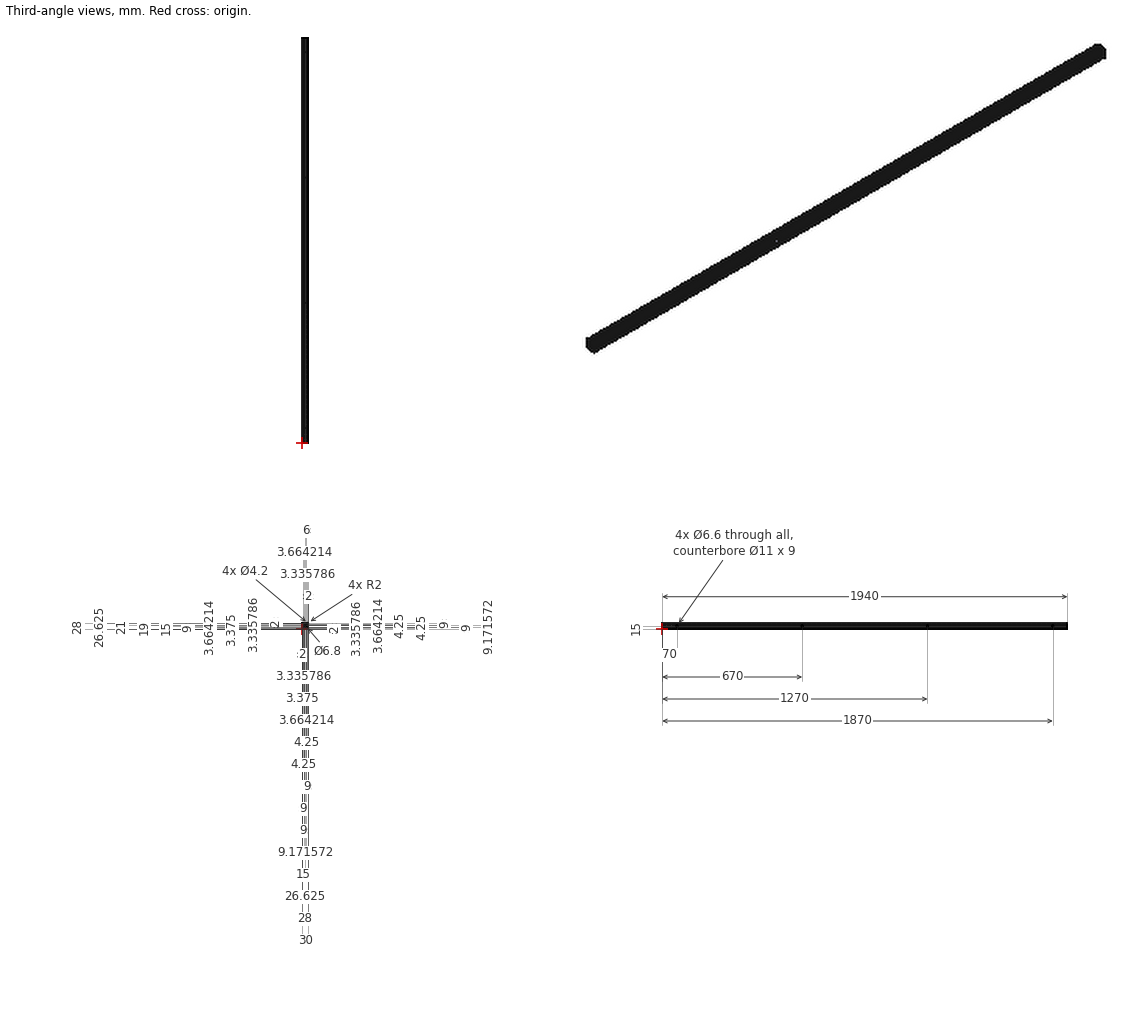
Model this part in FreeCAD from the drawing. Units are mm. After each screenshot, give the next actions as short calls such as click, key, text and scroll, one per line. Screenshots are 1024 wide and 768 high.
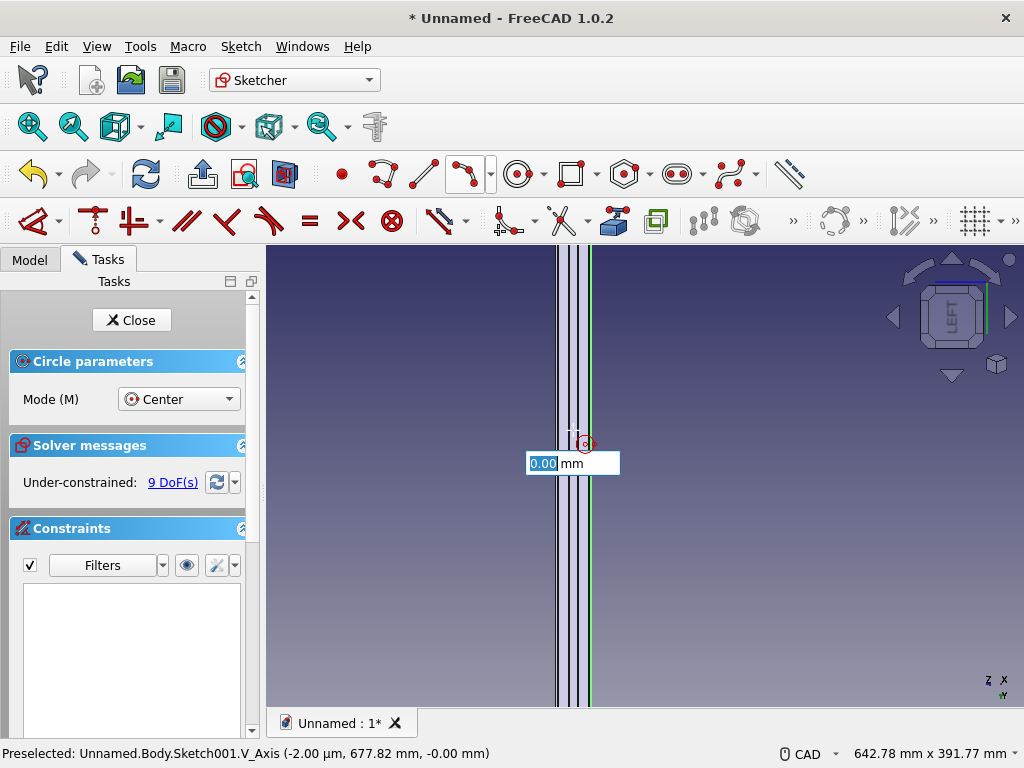
scroll(576, 427, up, 8)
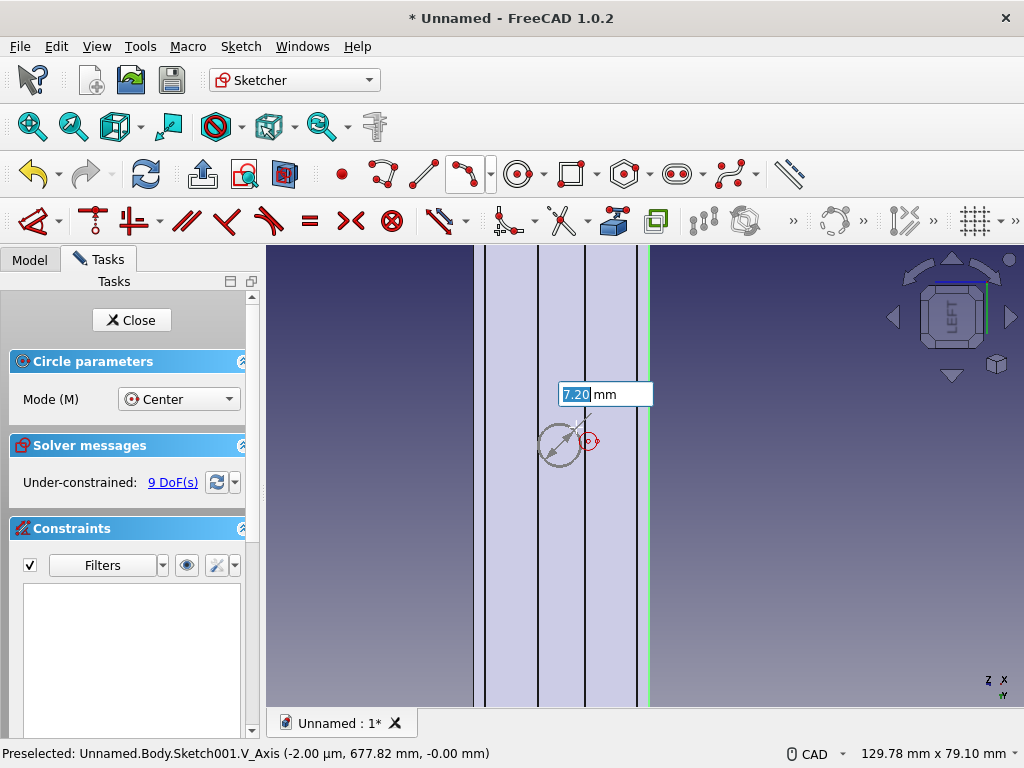
click(575, 424)
key(Escape)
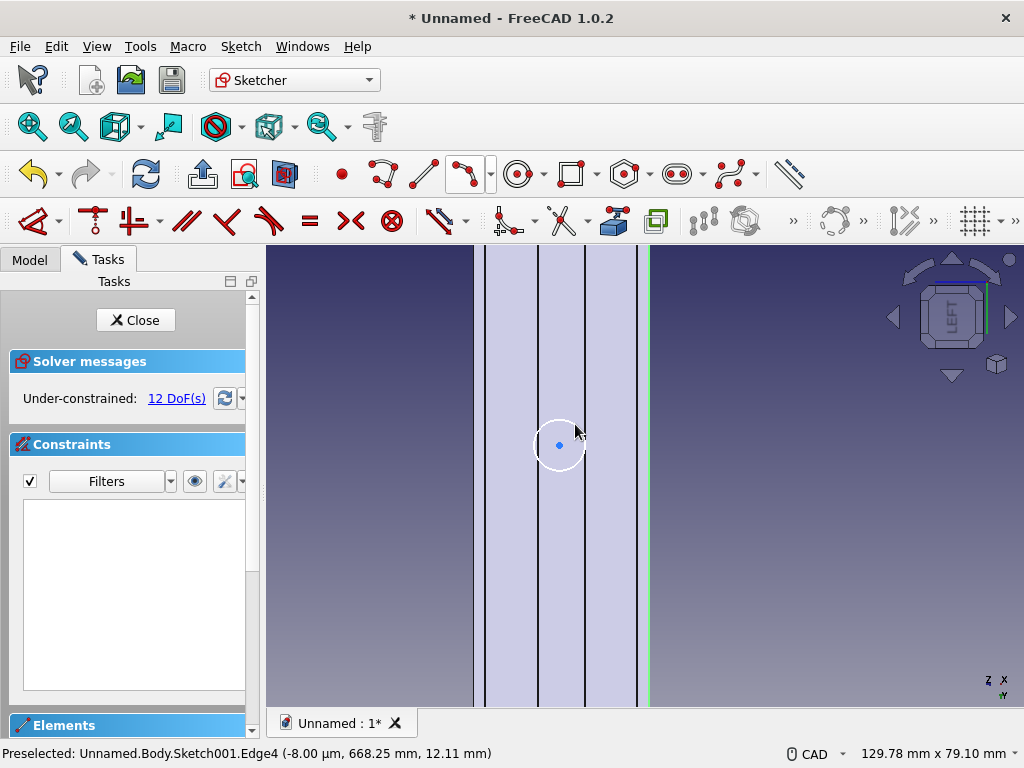
scroll(576, 433, down, 18)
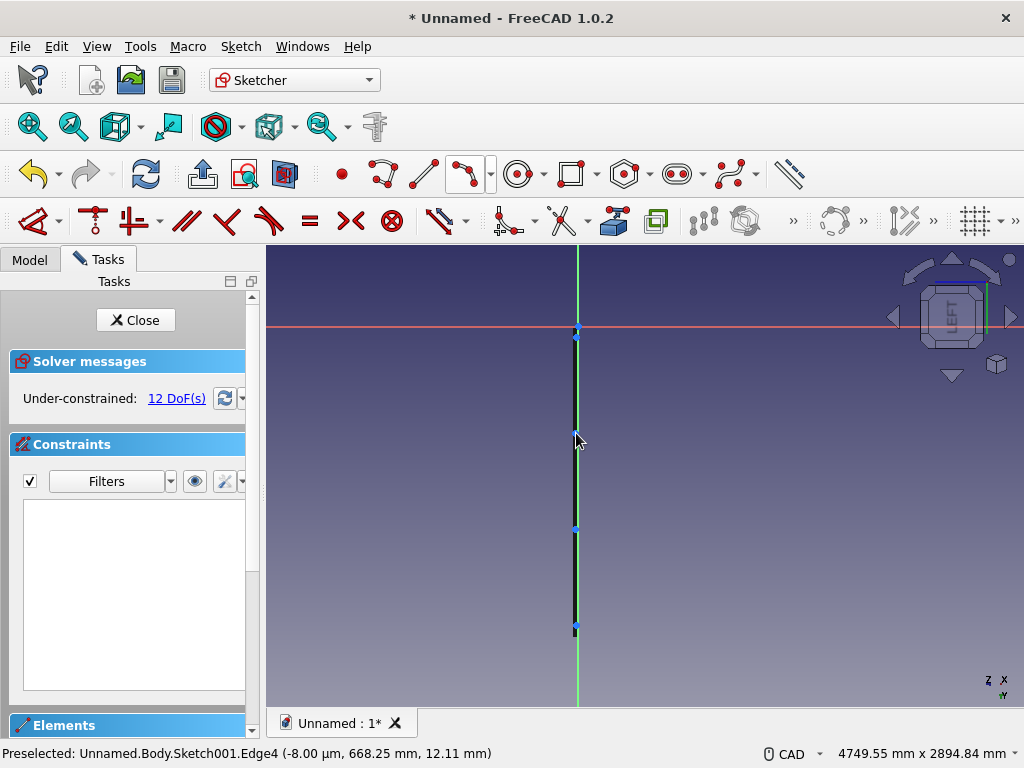
scroll(576, 337, up, 14)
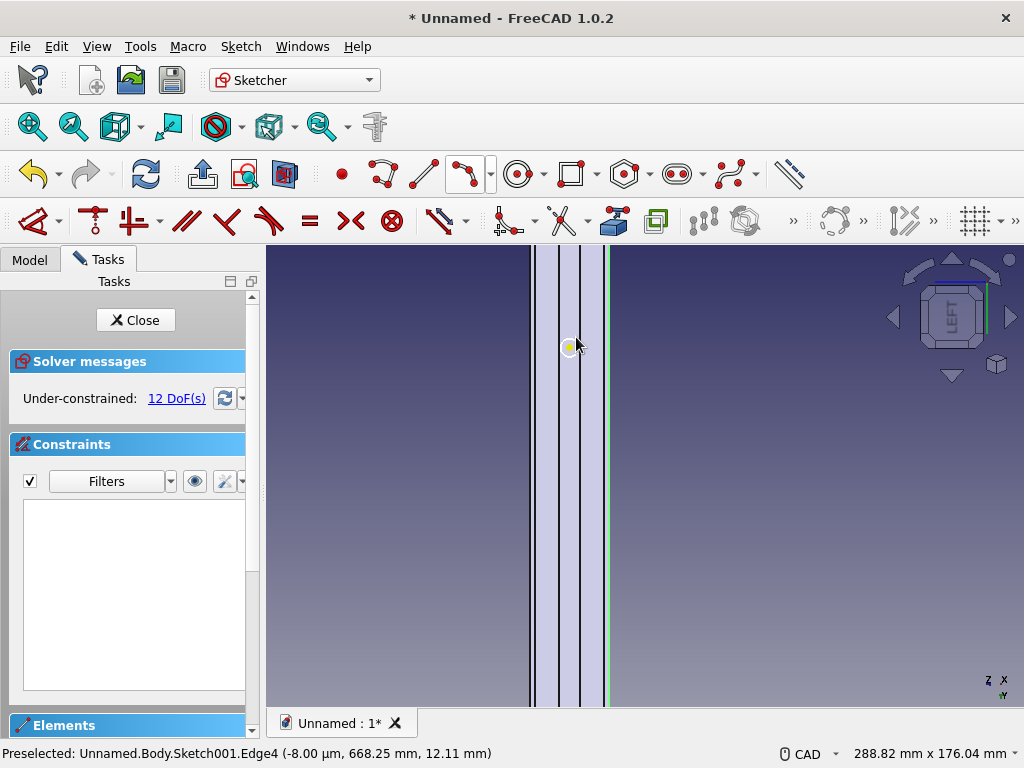
click(576, 341)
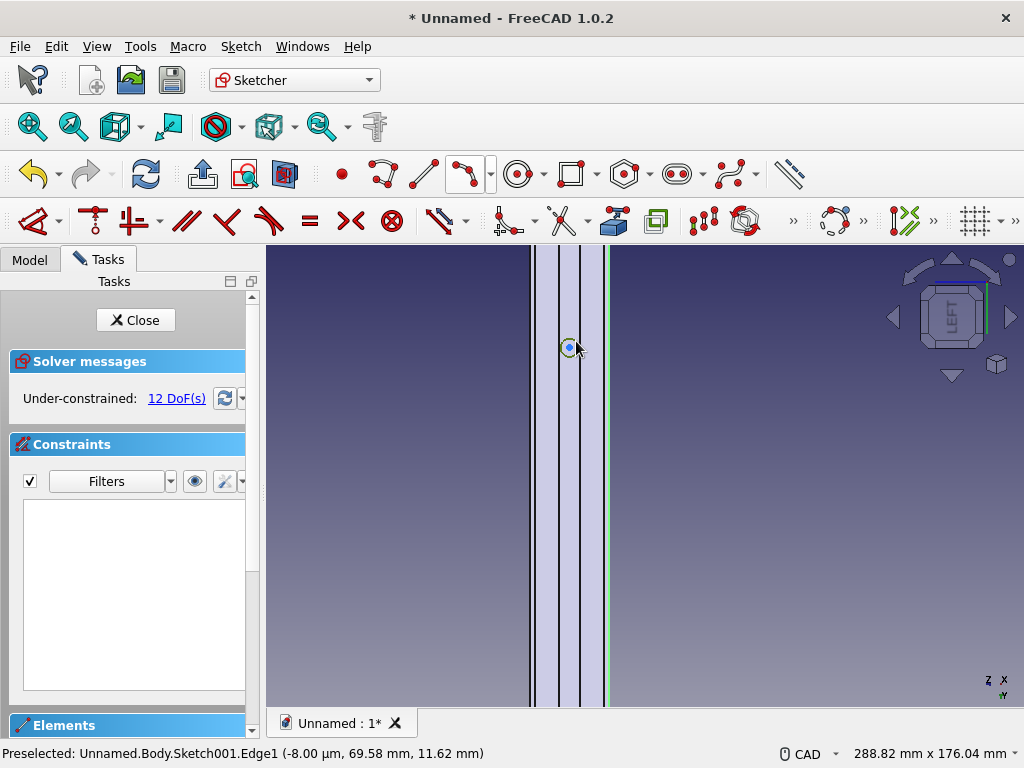
scroll(576, 337, down, 14)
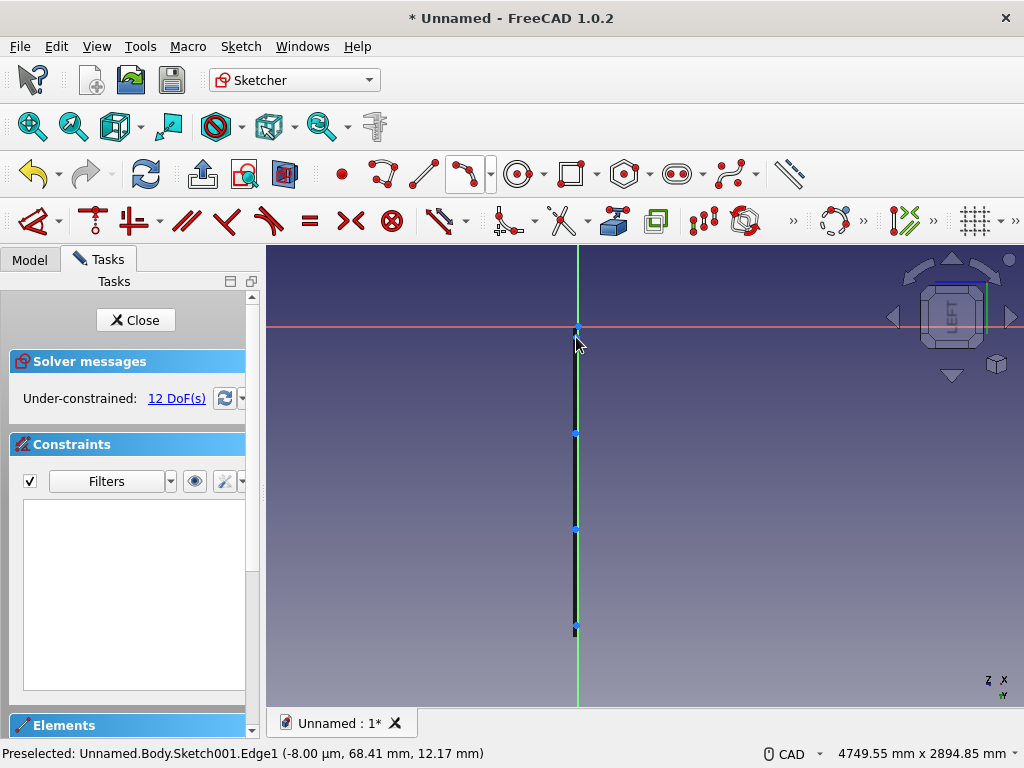
scroll(576, 625, up, 14)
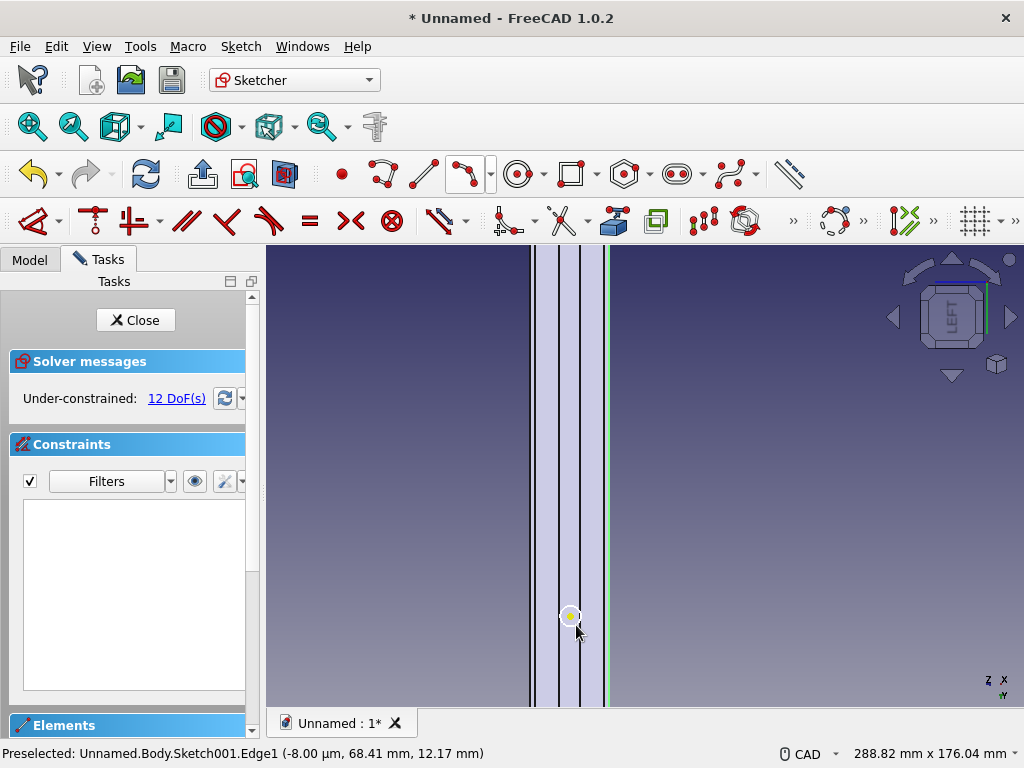
click(578, 609)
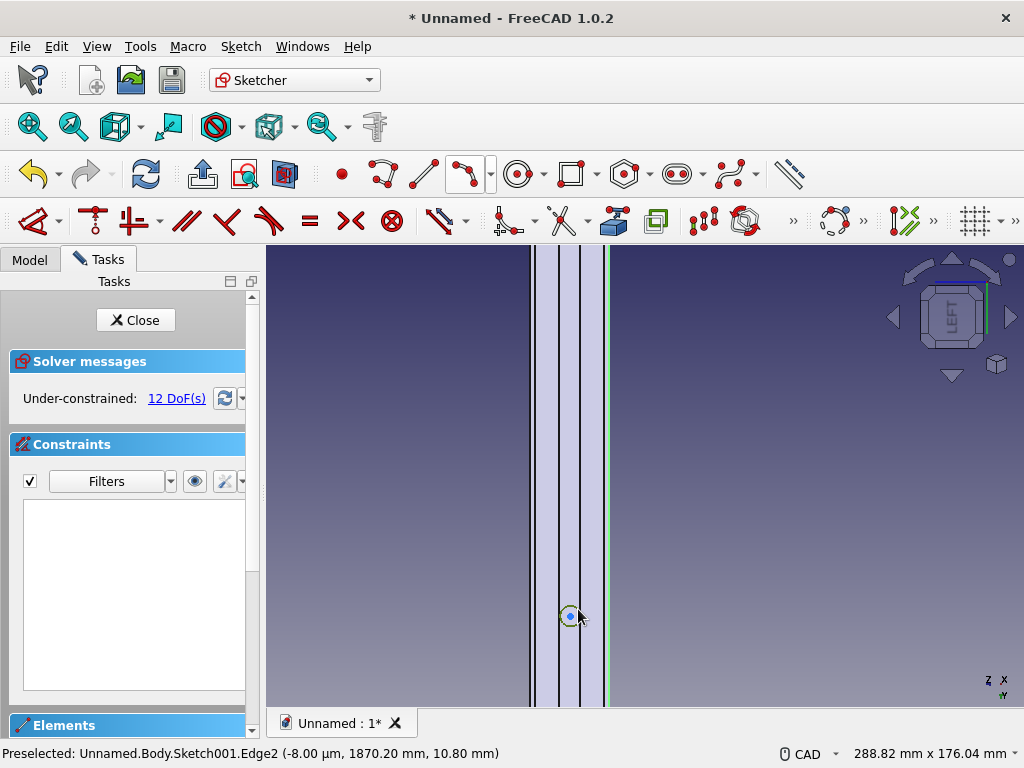
scroll(576, 626, down, 14)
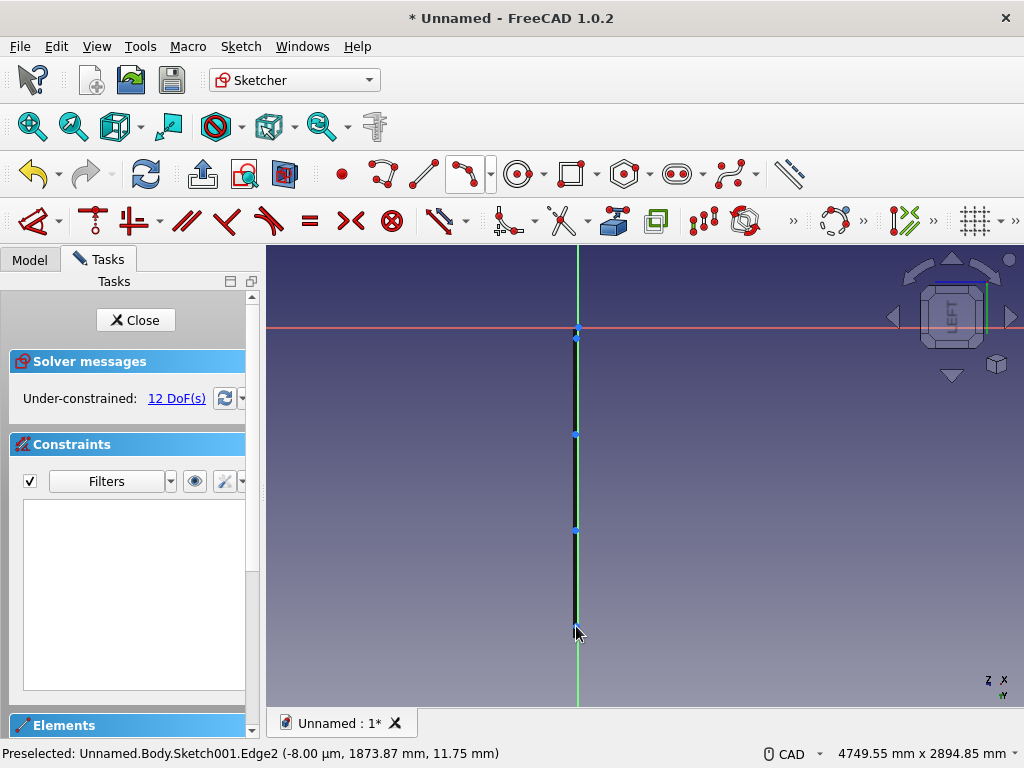
scroll(576, 530, up, 14)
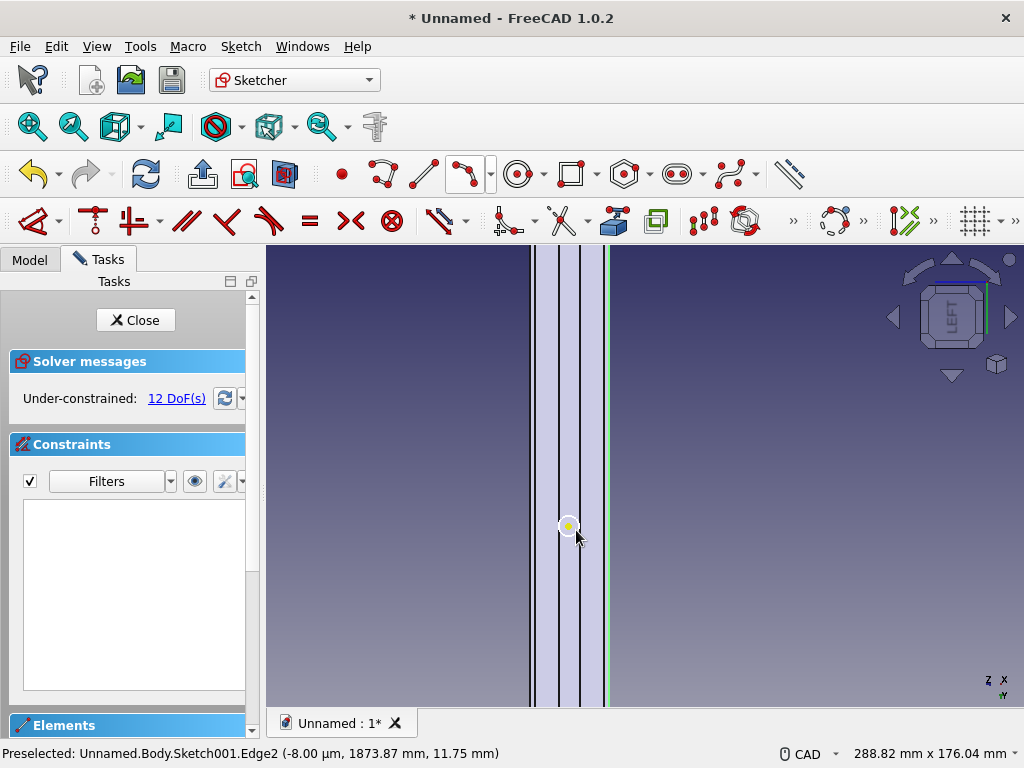
click(576, 519)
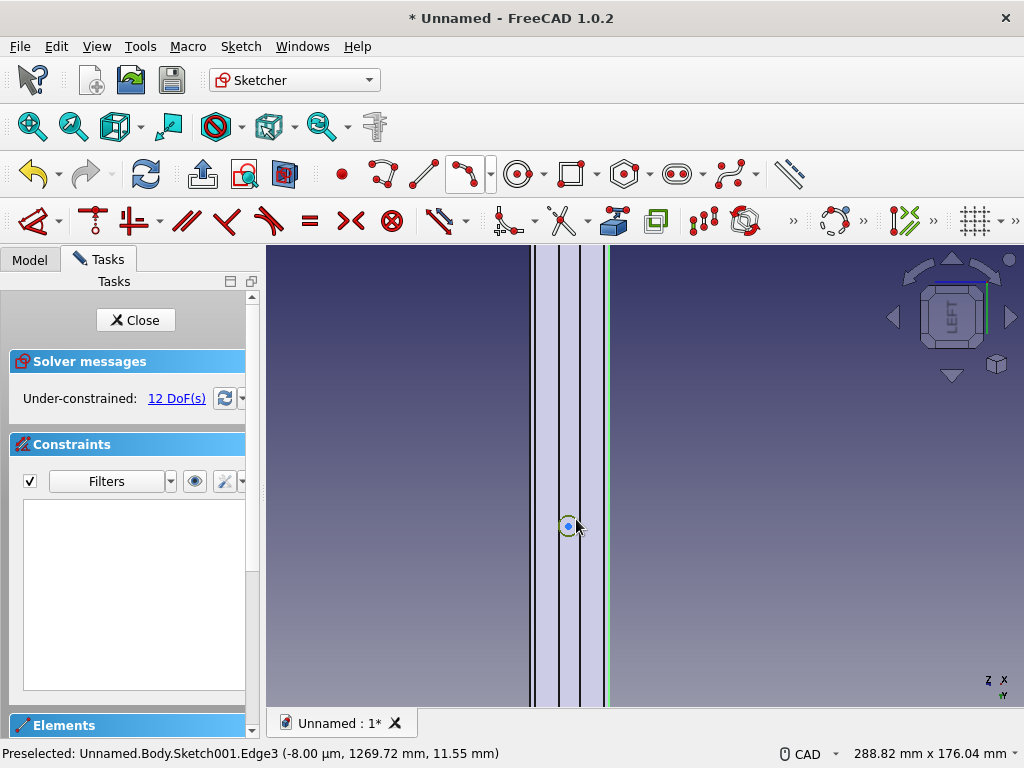
scroll(576, 530, down, 14)